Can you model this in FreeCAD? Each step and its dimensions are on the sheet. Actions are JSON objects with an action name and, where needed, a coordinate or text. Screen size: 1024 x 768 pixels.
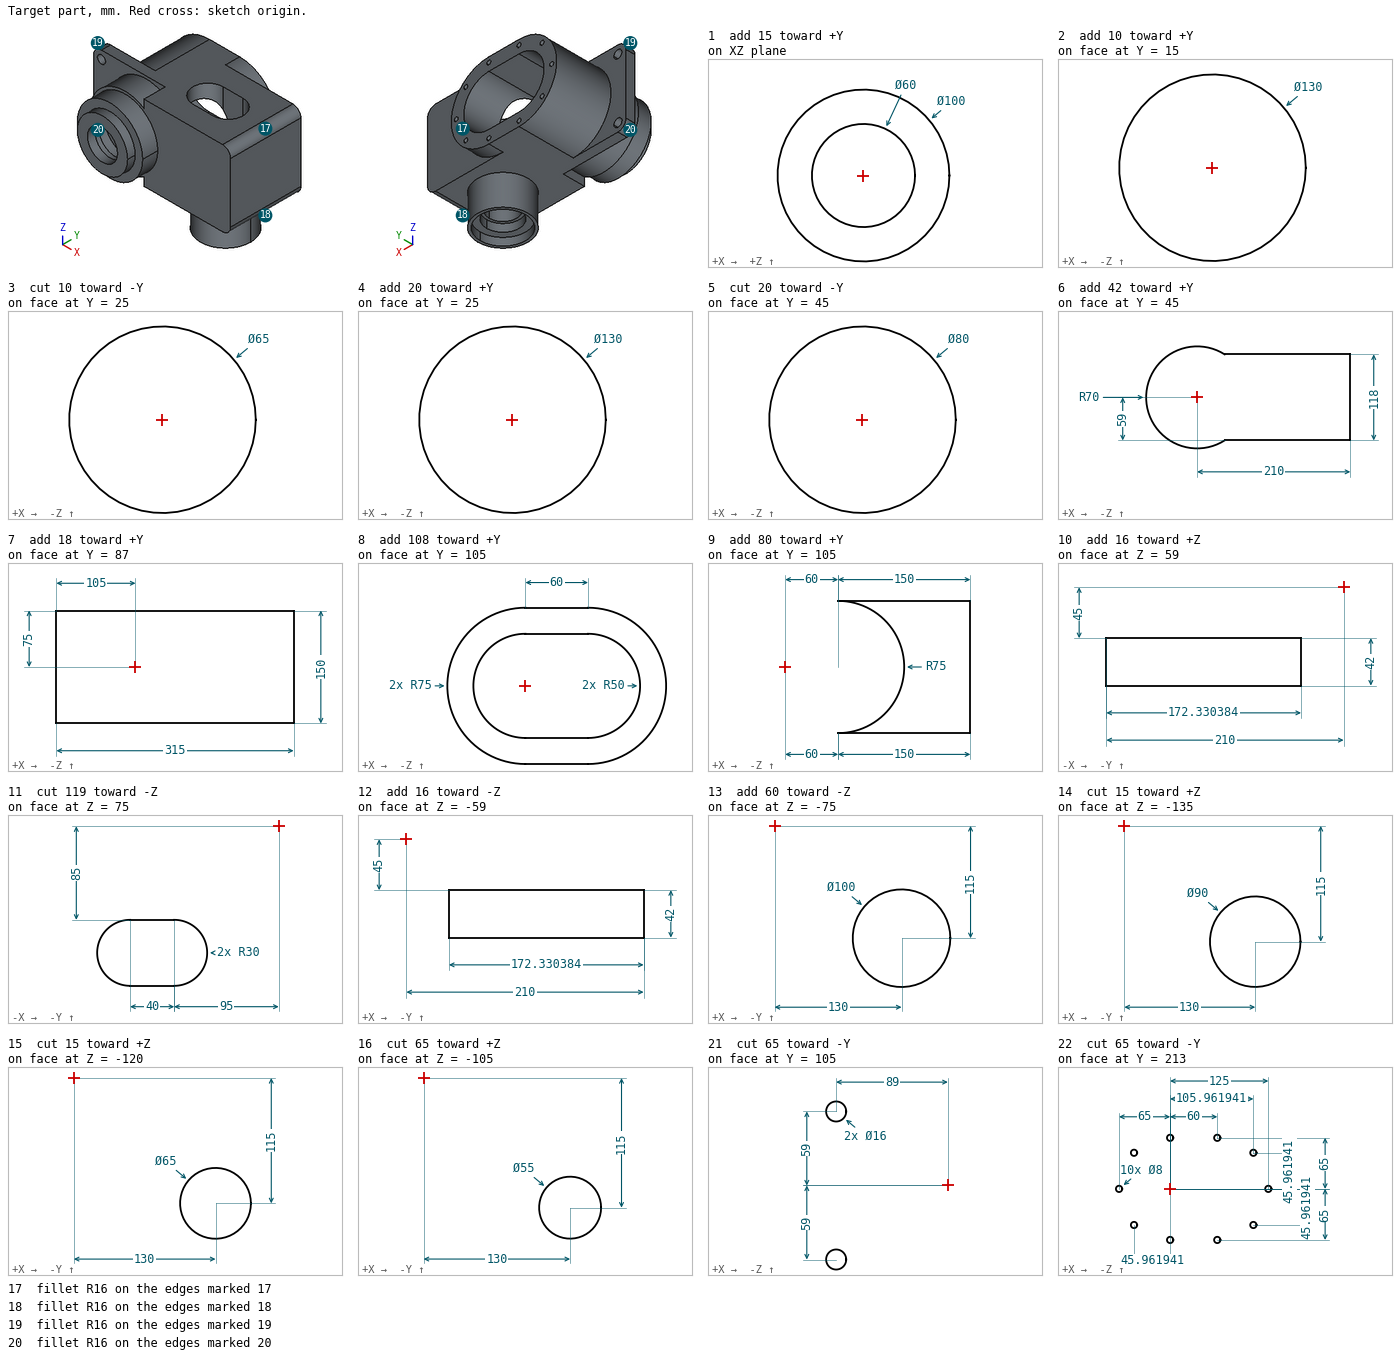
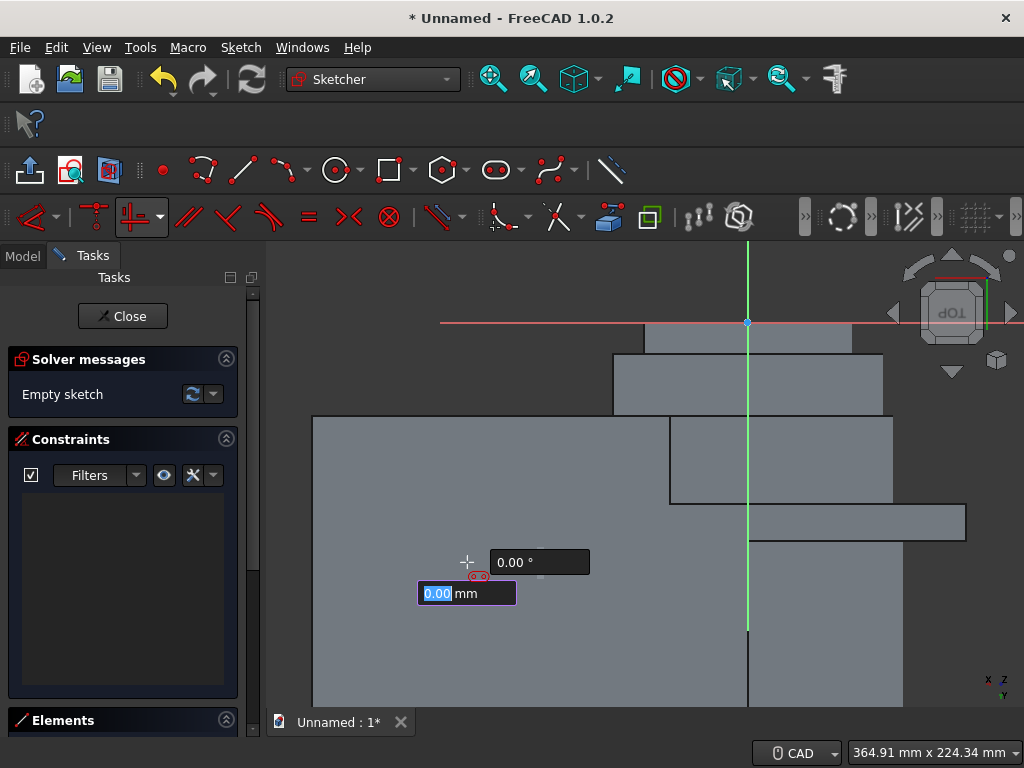
{"action": "left_click", "coordinate": [551, 562]}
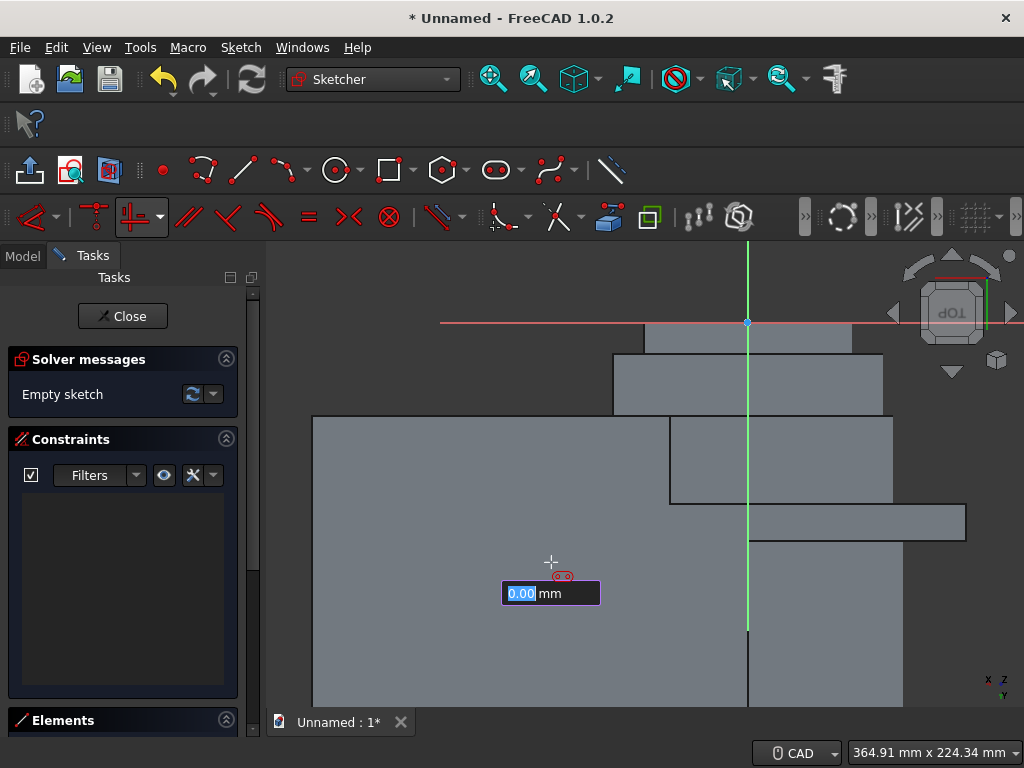
{"action": "left_click", "coordinate": [509, 624]}
{"action": "key", "text": "Escape"}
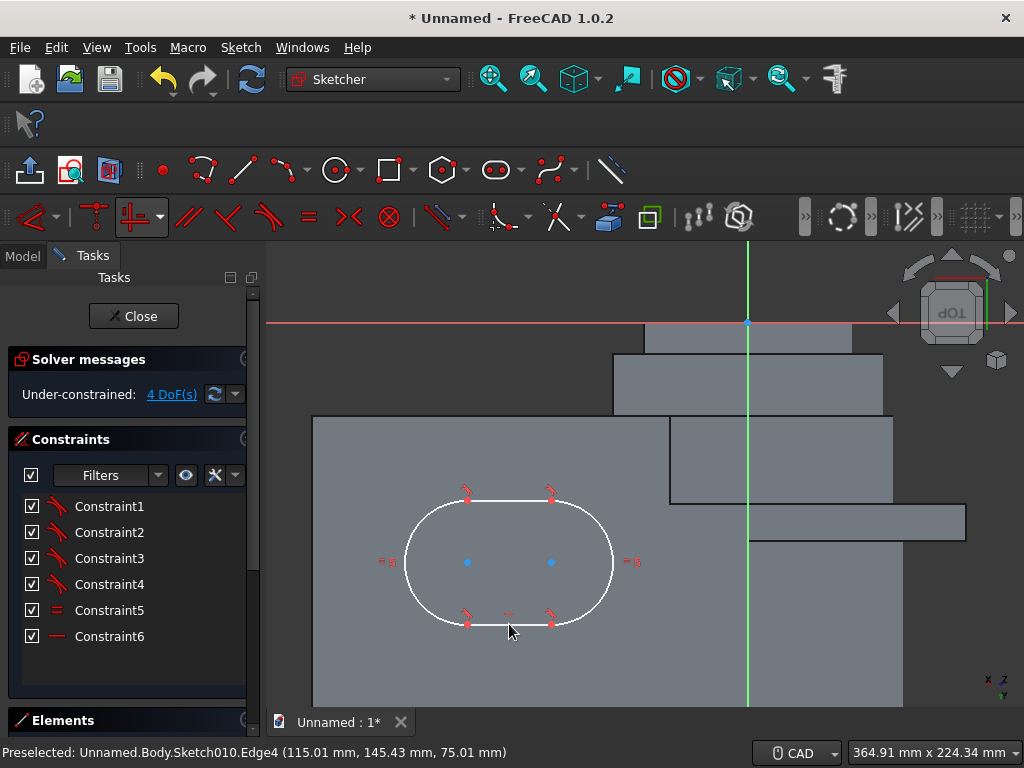
{"action": "left_click", "coordinate": [32, 218]}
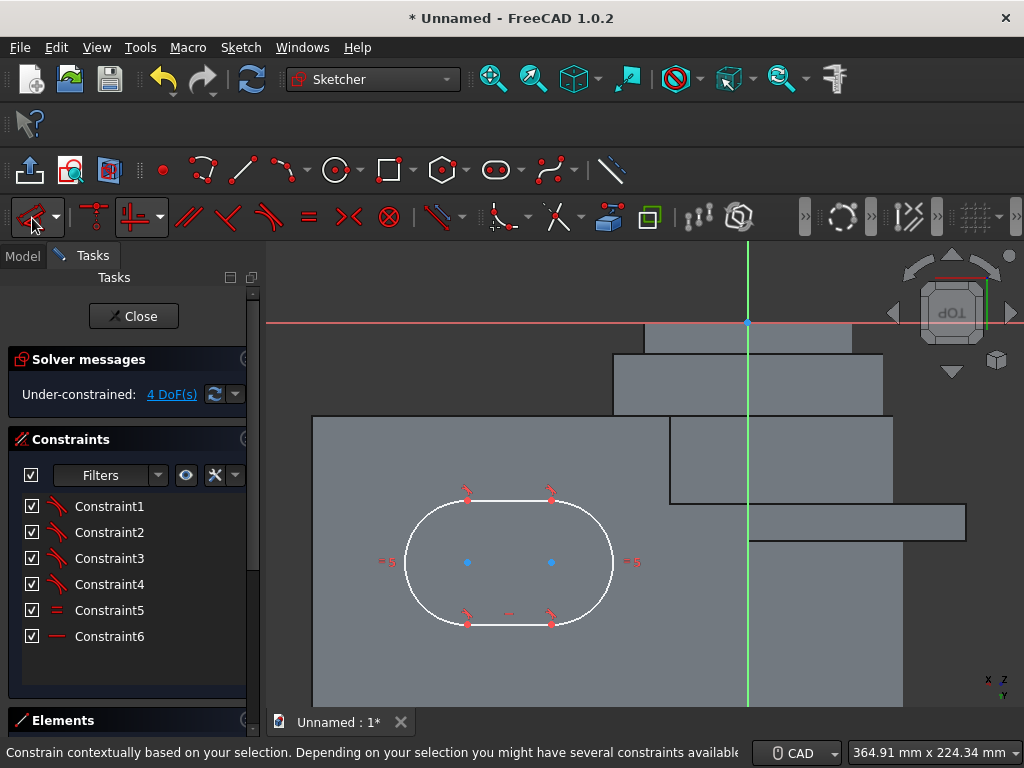
{"action": "left_click", "coordinate": [417, 527]}
{"action": "left_click", "coordinate": [391, 508]}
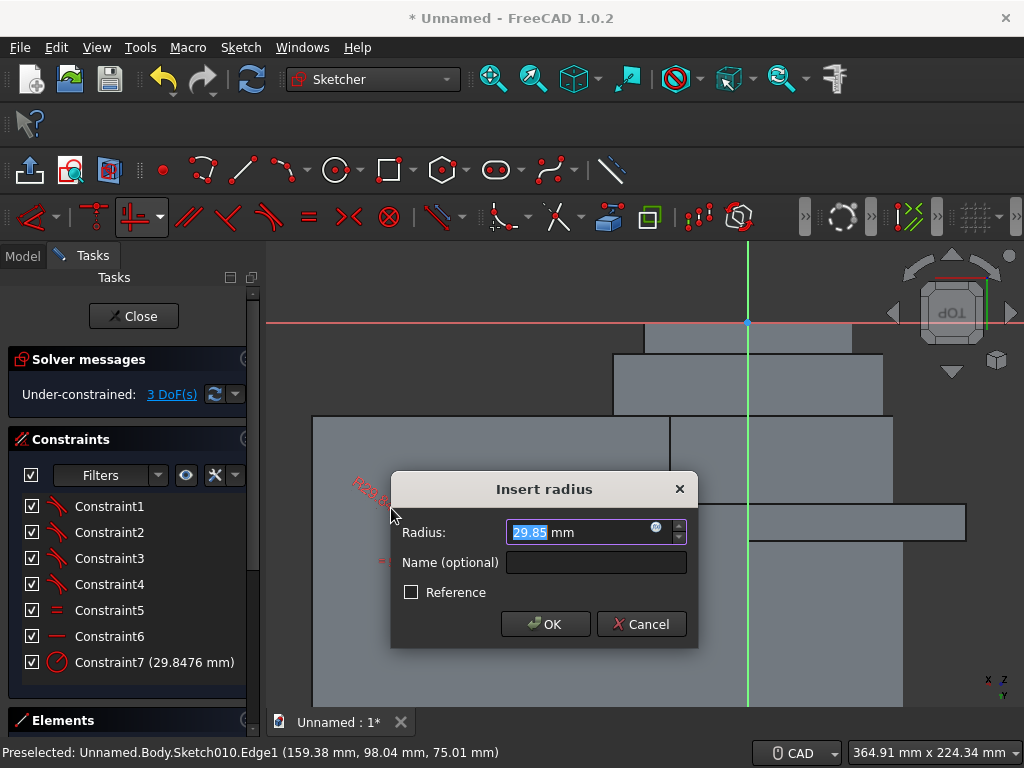
{"action": "type", "text": "30"}
{"action": "key", "text": "Return"}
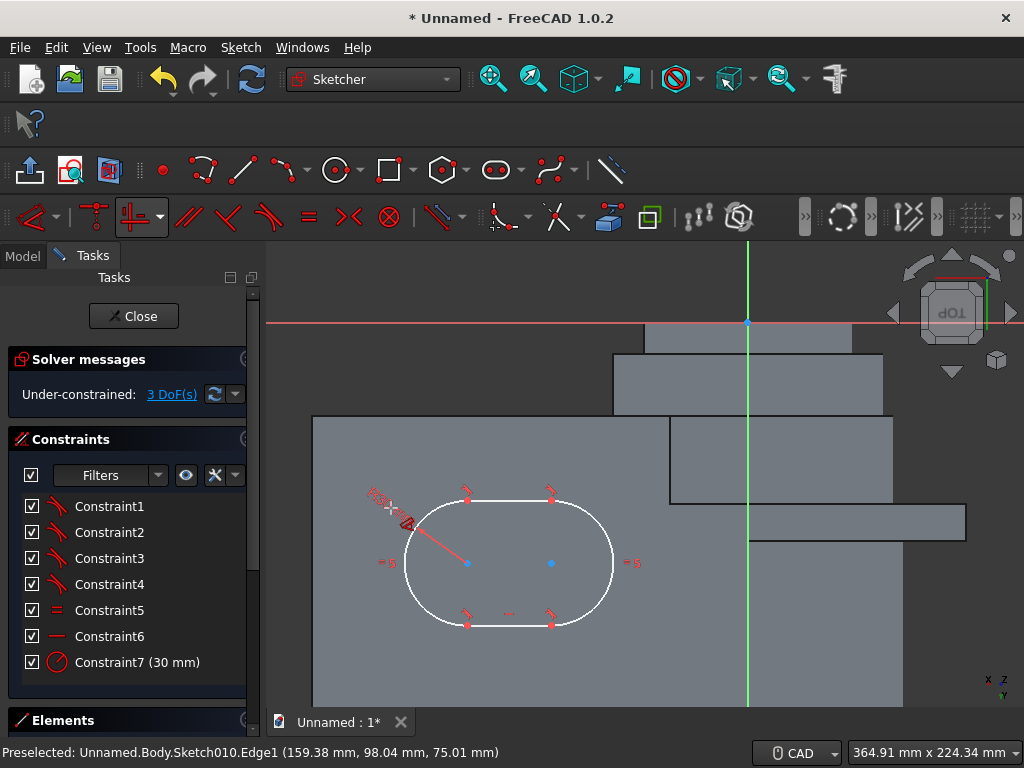
{"action": "left_click", "coordinate": [492, 501]}
{"action": "left_click", "coordinate": [509, 535]}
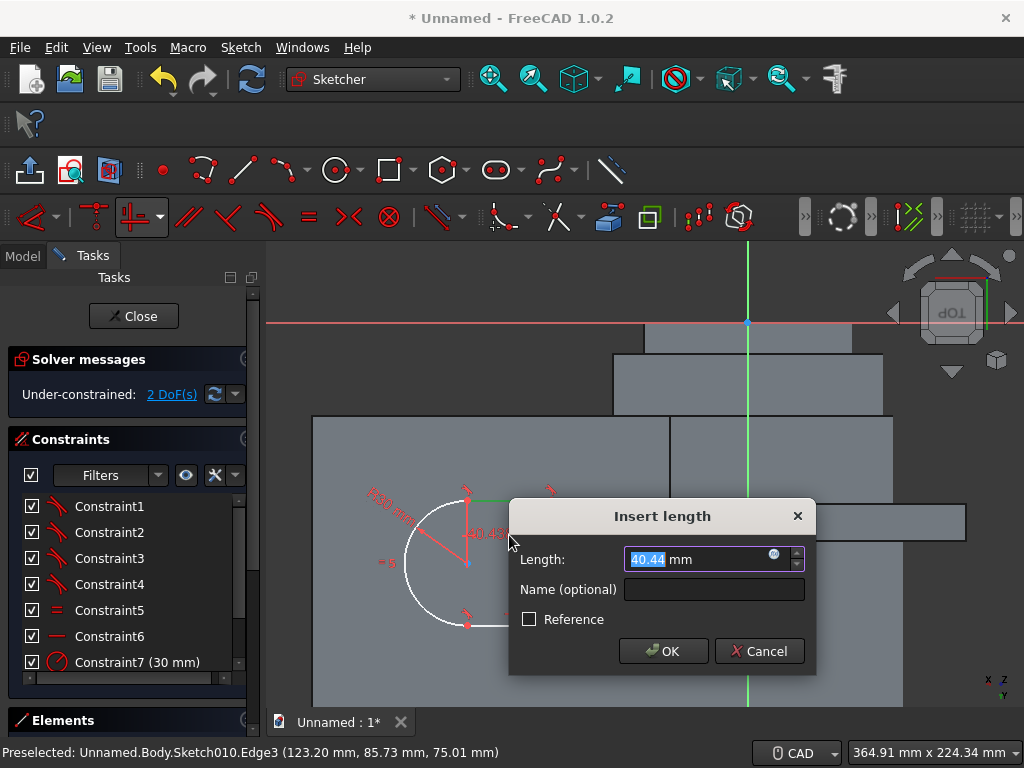
{"action": "type", "text": "40"}
{"action": "key", "text": "Return"}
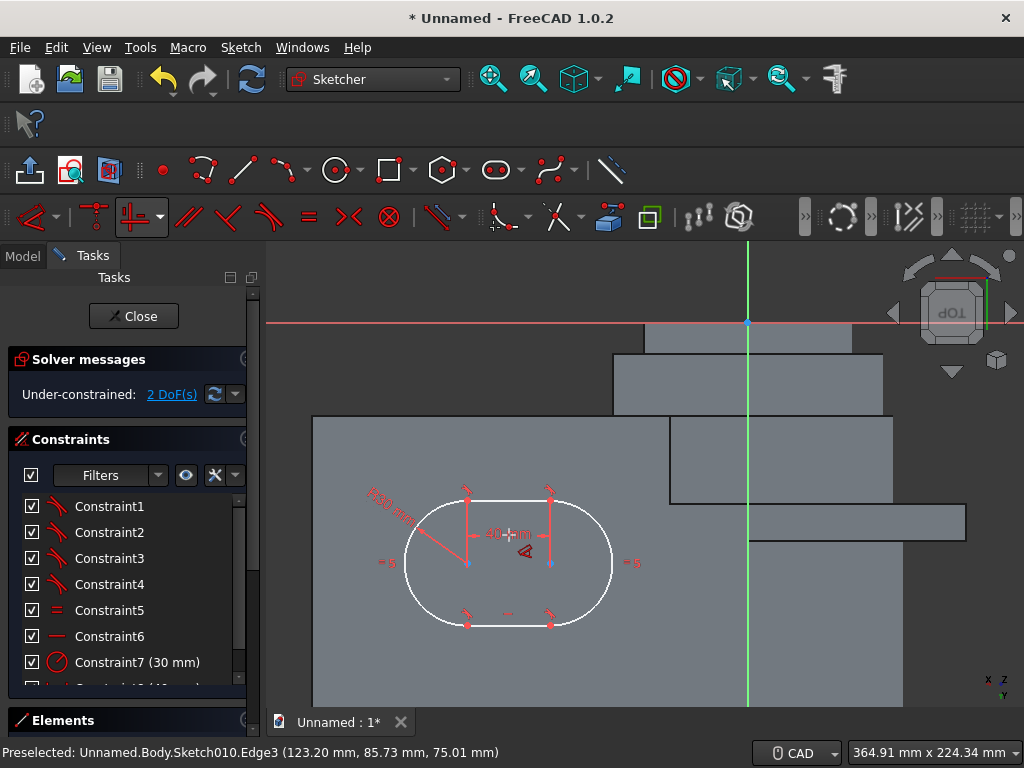
{"action": "left_click", "coordinate": [467, 501]}
{"action": "left_click", "coordinate": [782, 412]}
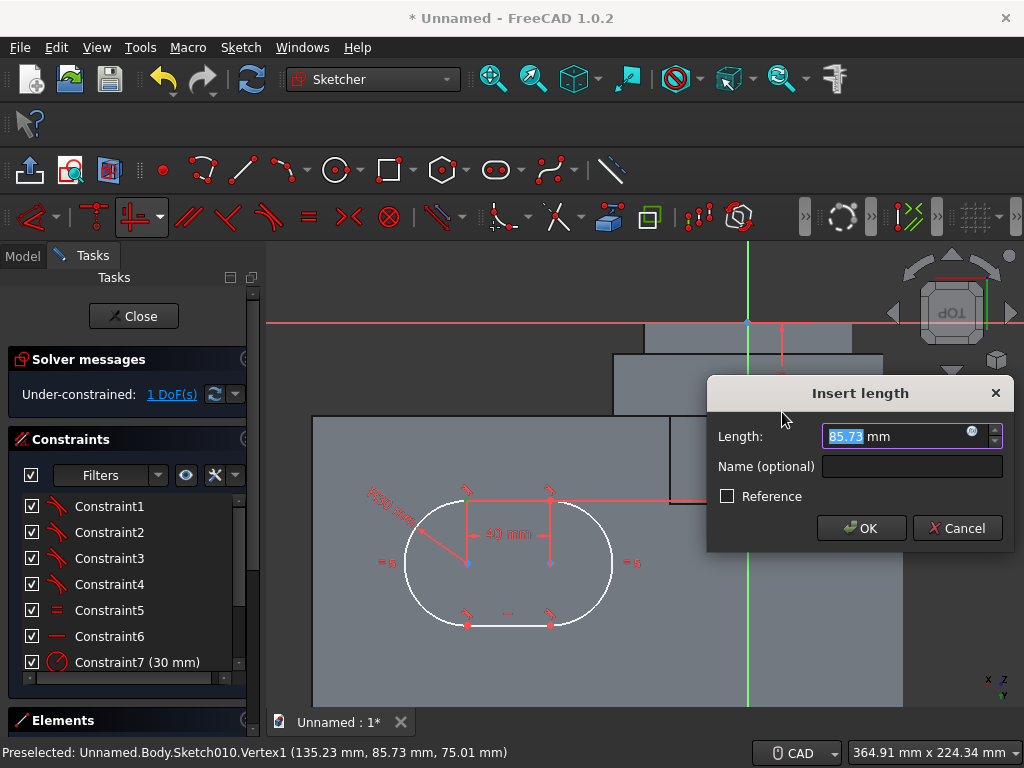
{"action": "type", "text": "85"}
{"action": "key", "text": "Return"}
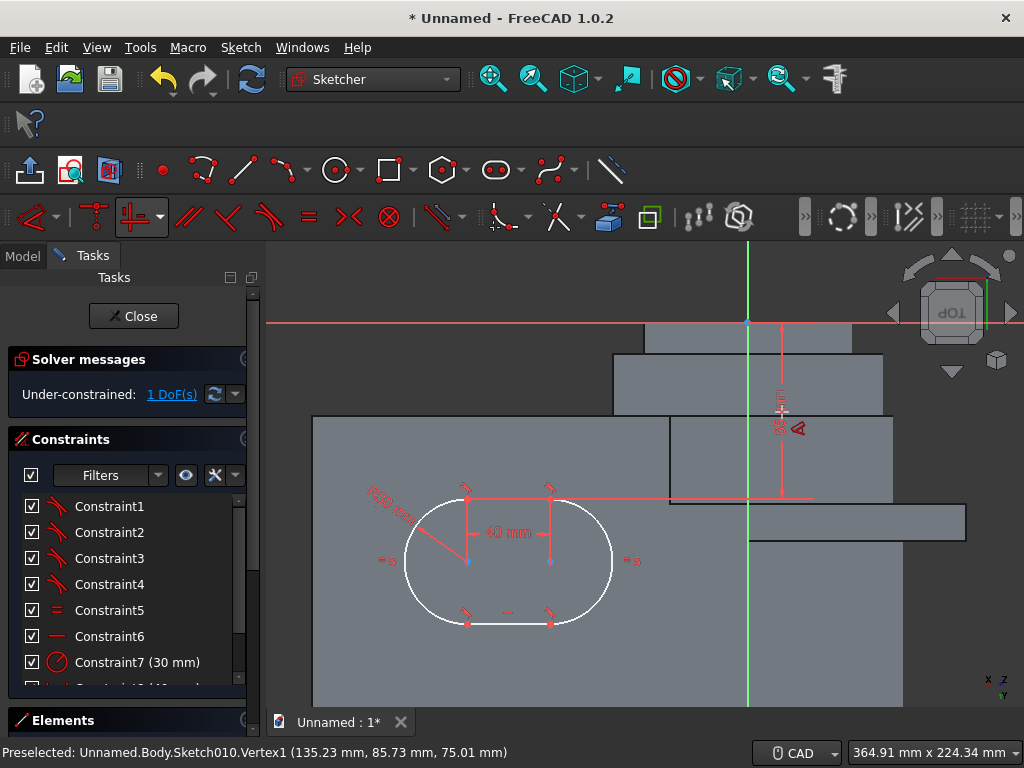
{"action": "left_click", "coordinate": [550, 624]}
{"action": "left_click", "coordinate": [649, 658]}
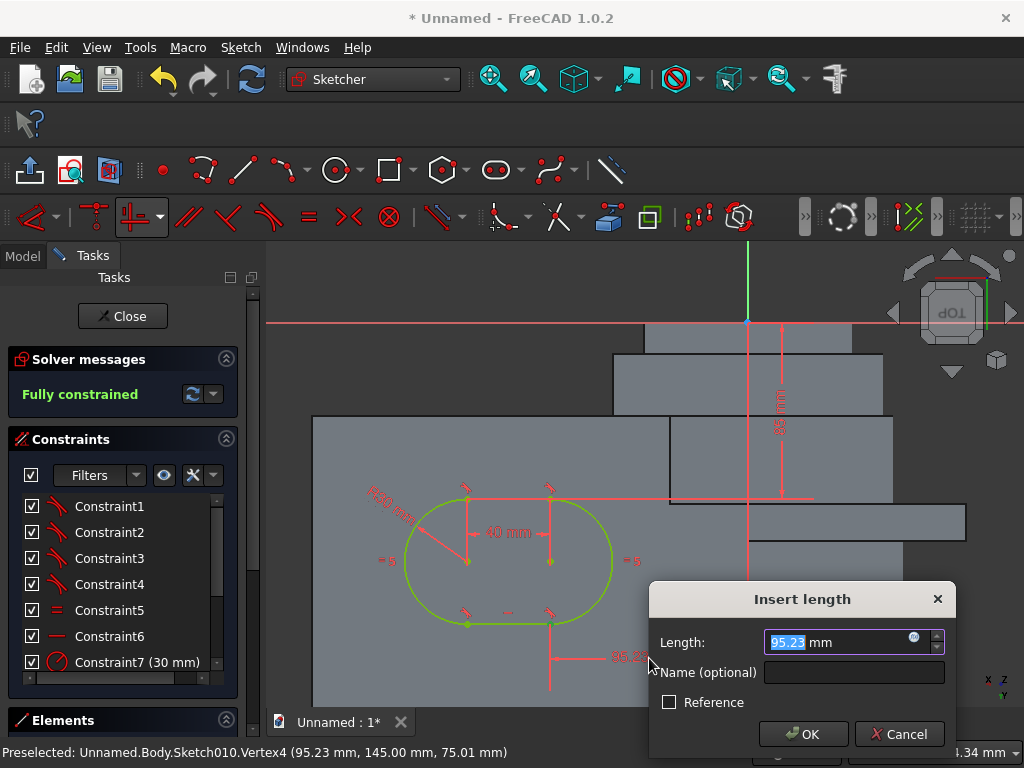
{"action": "type", "text": "95"}
{"action": "key", "text": "Return"}
{"action": "key", "text": "Escape"}